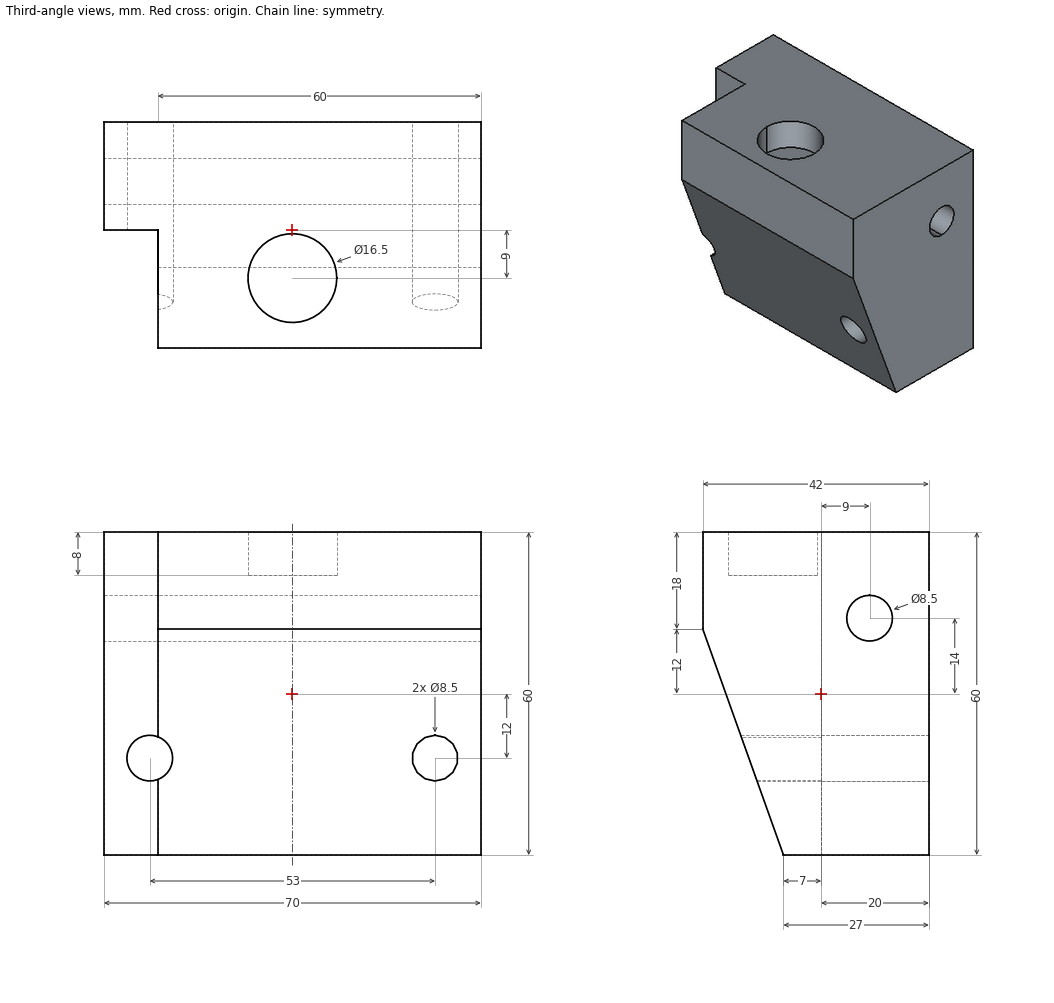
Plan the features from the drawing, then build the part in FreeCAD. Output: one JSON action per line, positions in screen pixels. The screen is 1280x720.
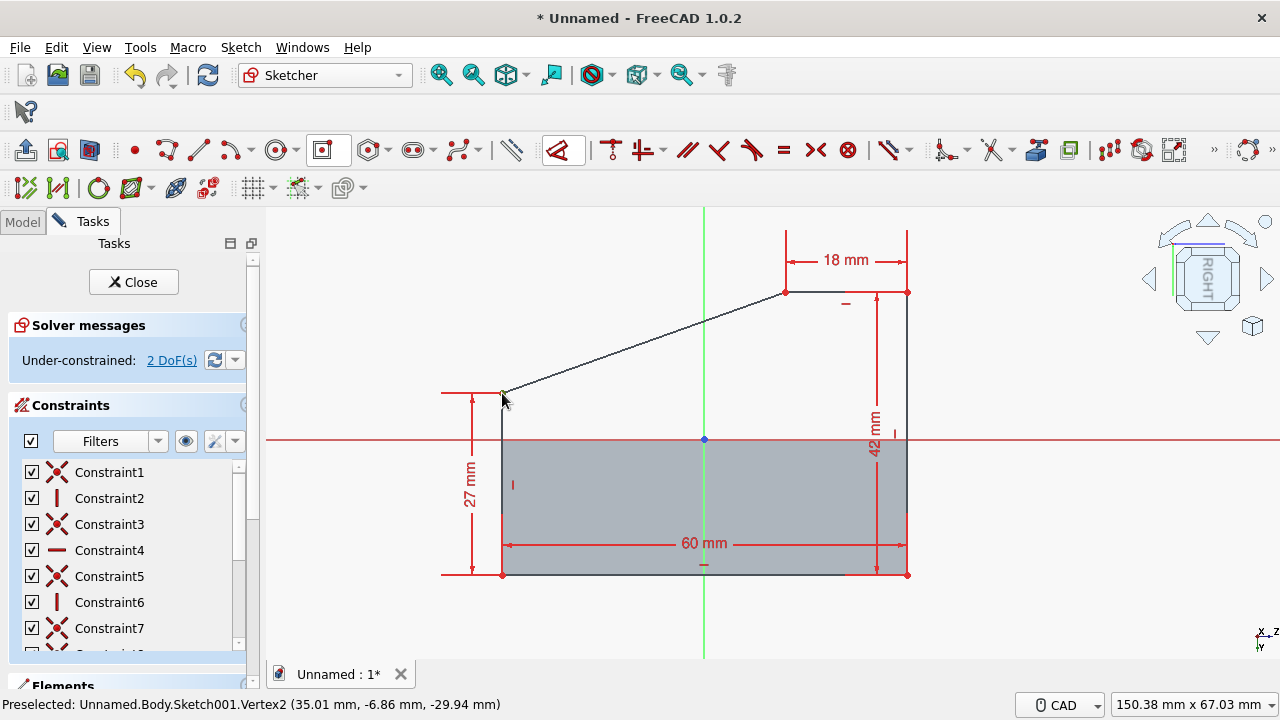
{"action": "key", "text": "i"}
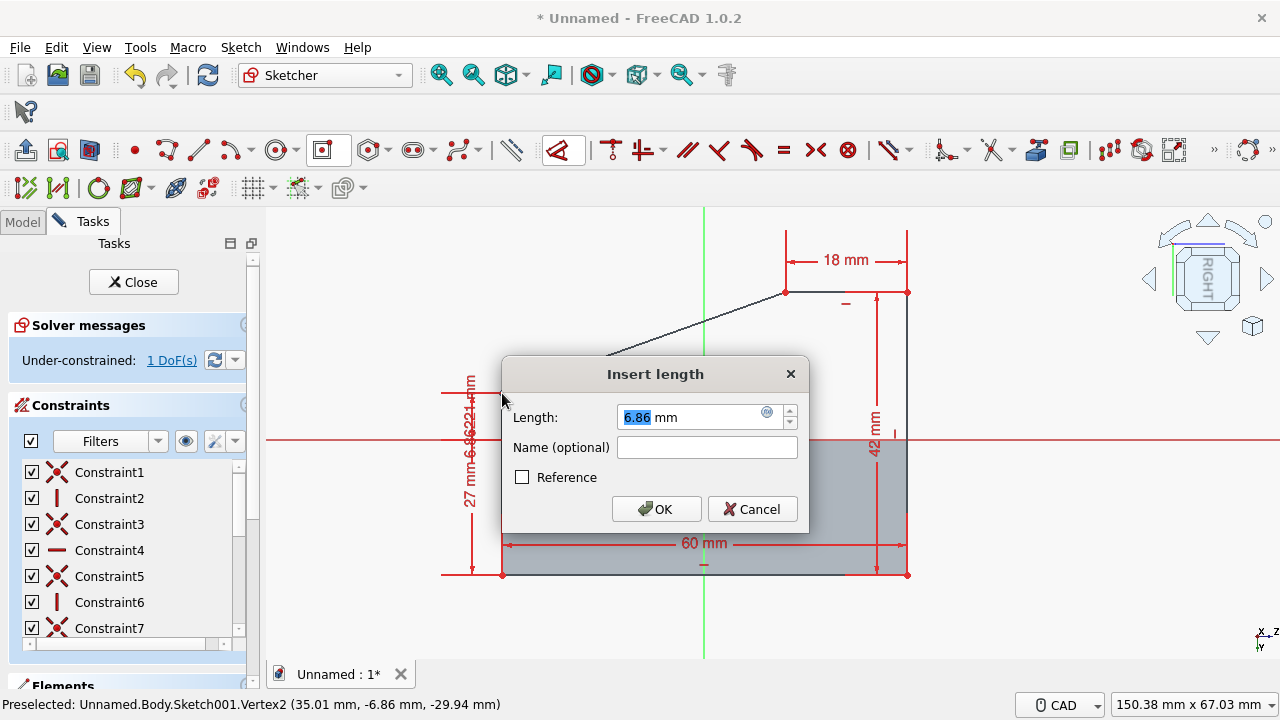
{"action": "type", "text": "7"}
{"action": "key", "text": "Return"}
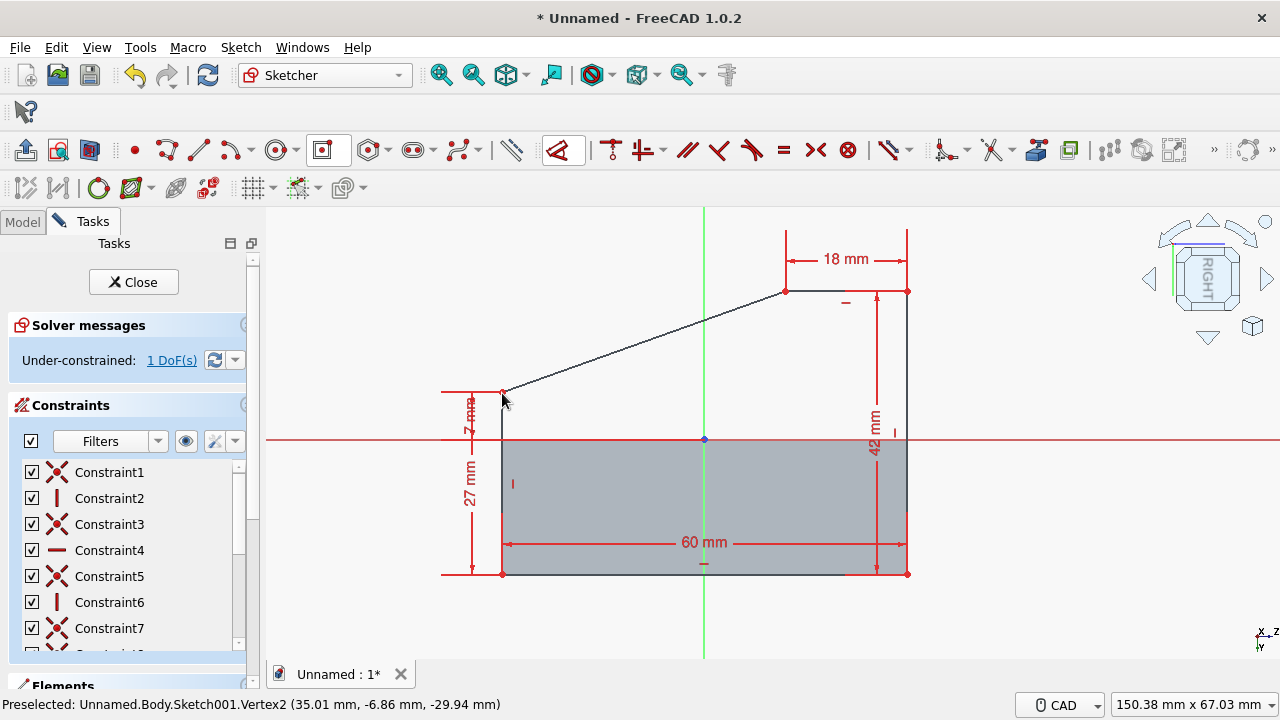
{"action": "left_click", "coordinate": [786, 291]}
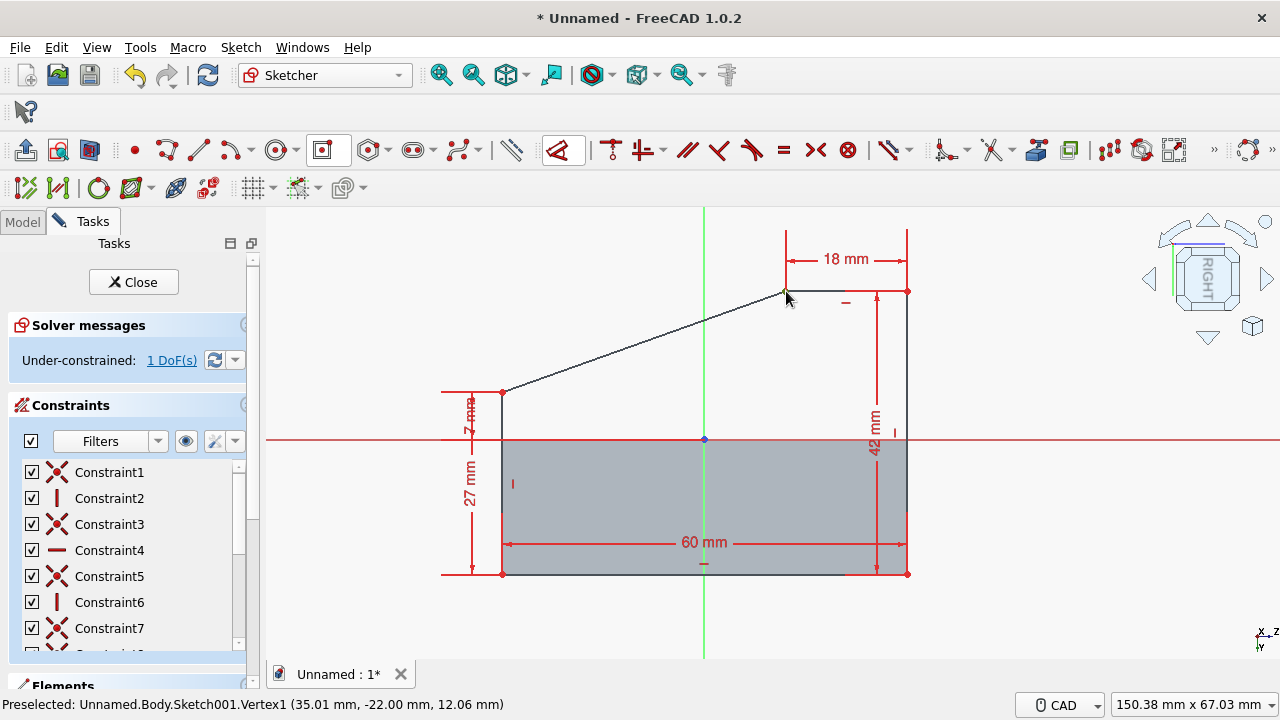
{"action": "left_click", "coordinate": [580, 150]}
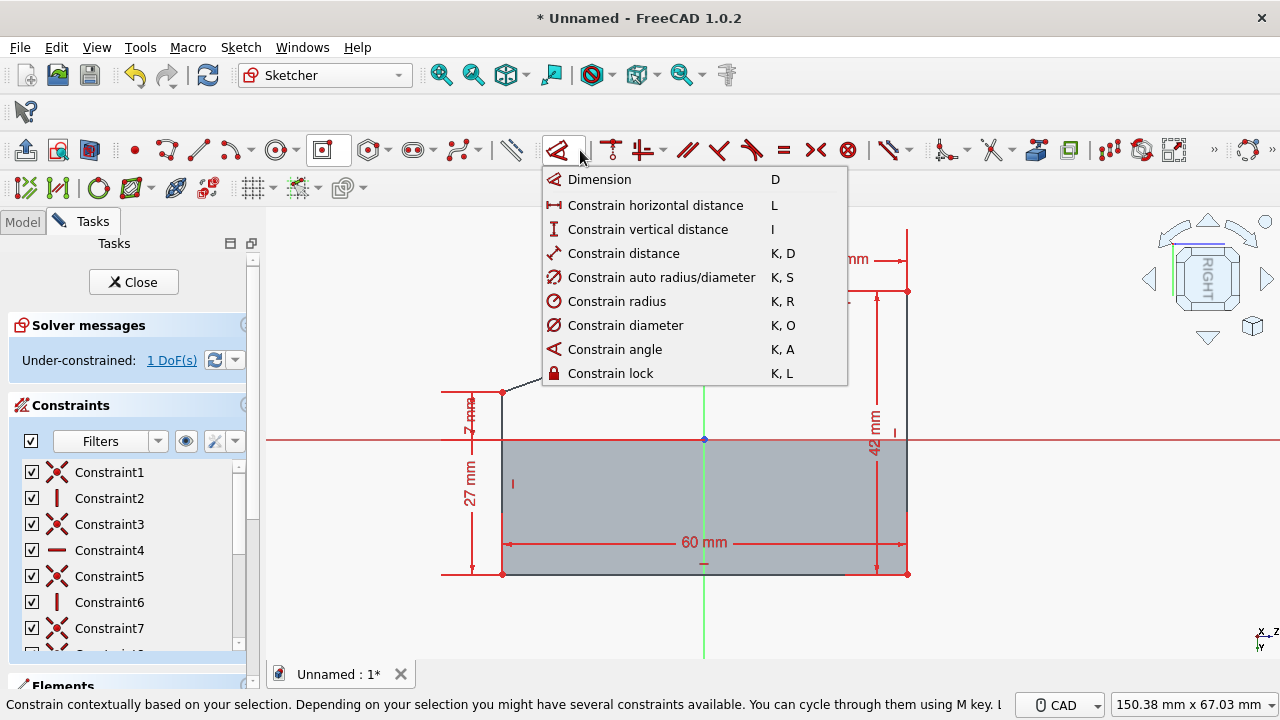
{"action": "left_click", "coordinate": [695, 205]}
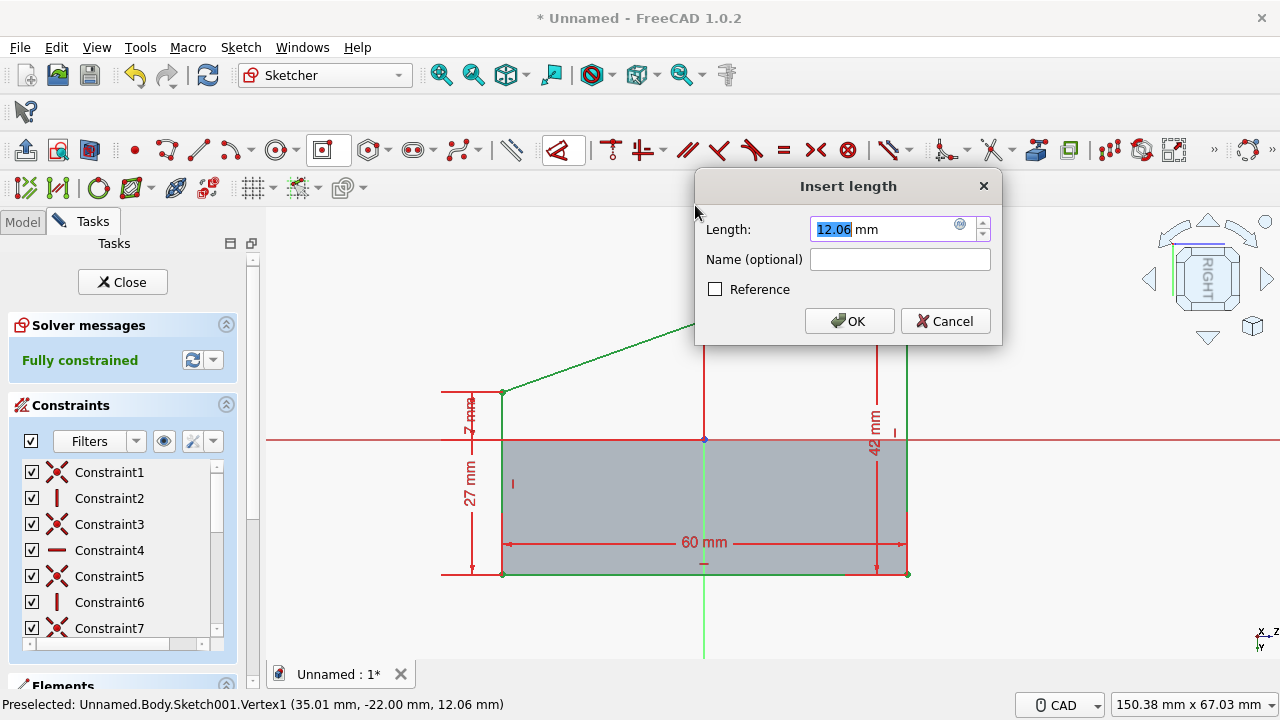
{"action": "type", "text": "12"}
{"action": "key", "text": "Return"}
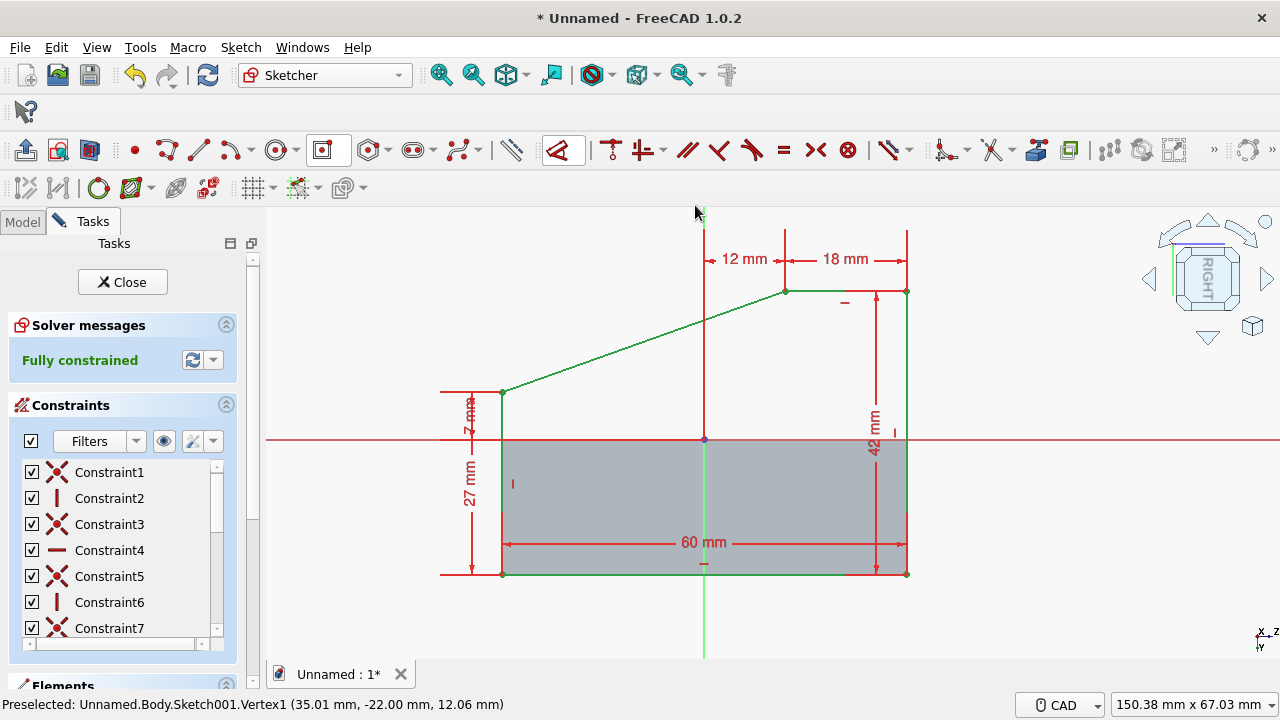
{"action": "left_click", "coordinate": [123, 282]}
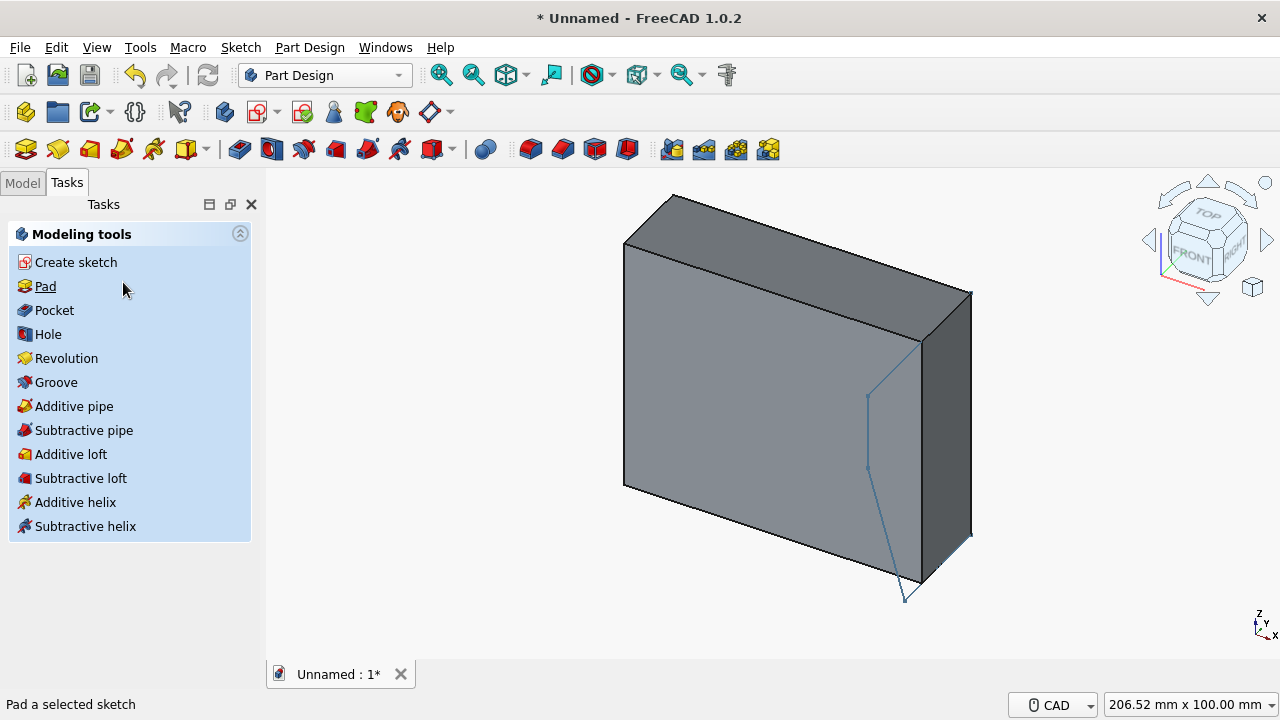
{"action": "left_click", "coordinate": [26, 150]}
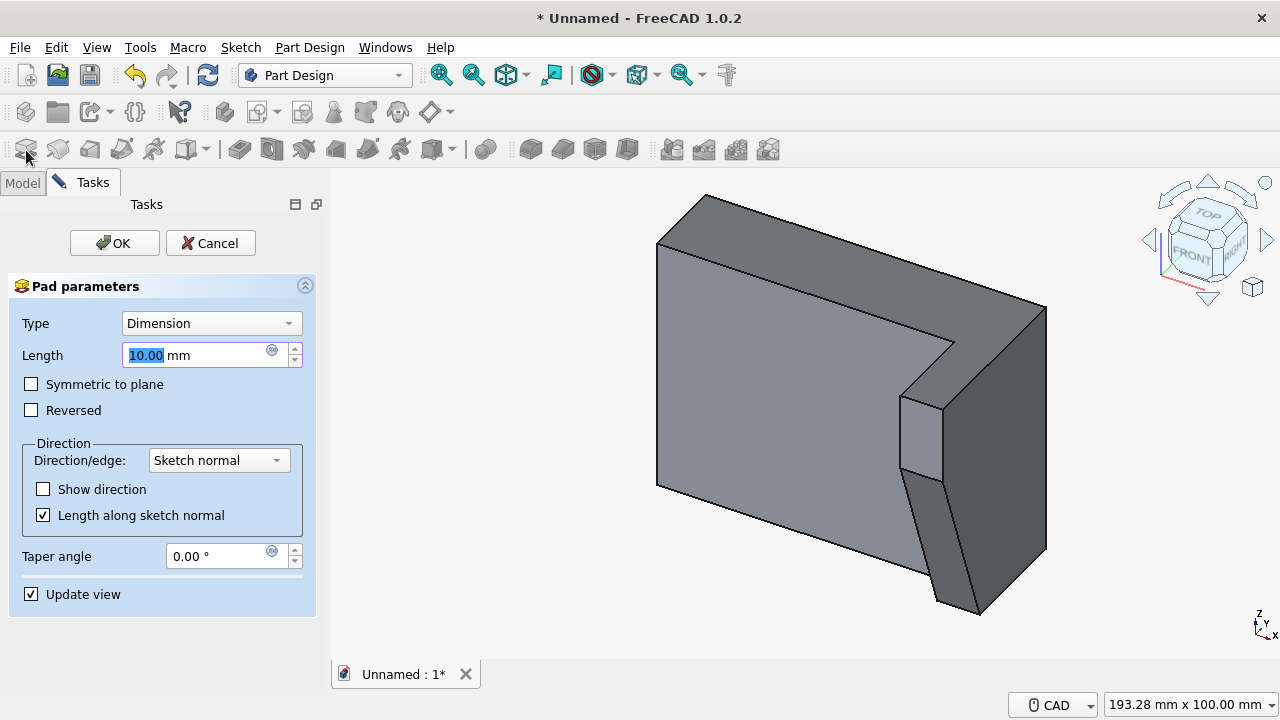
{"action": "type", "text": "60"}
{"action": "key", "text": "Tab"}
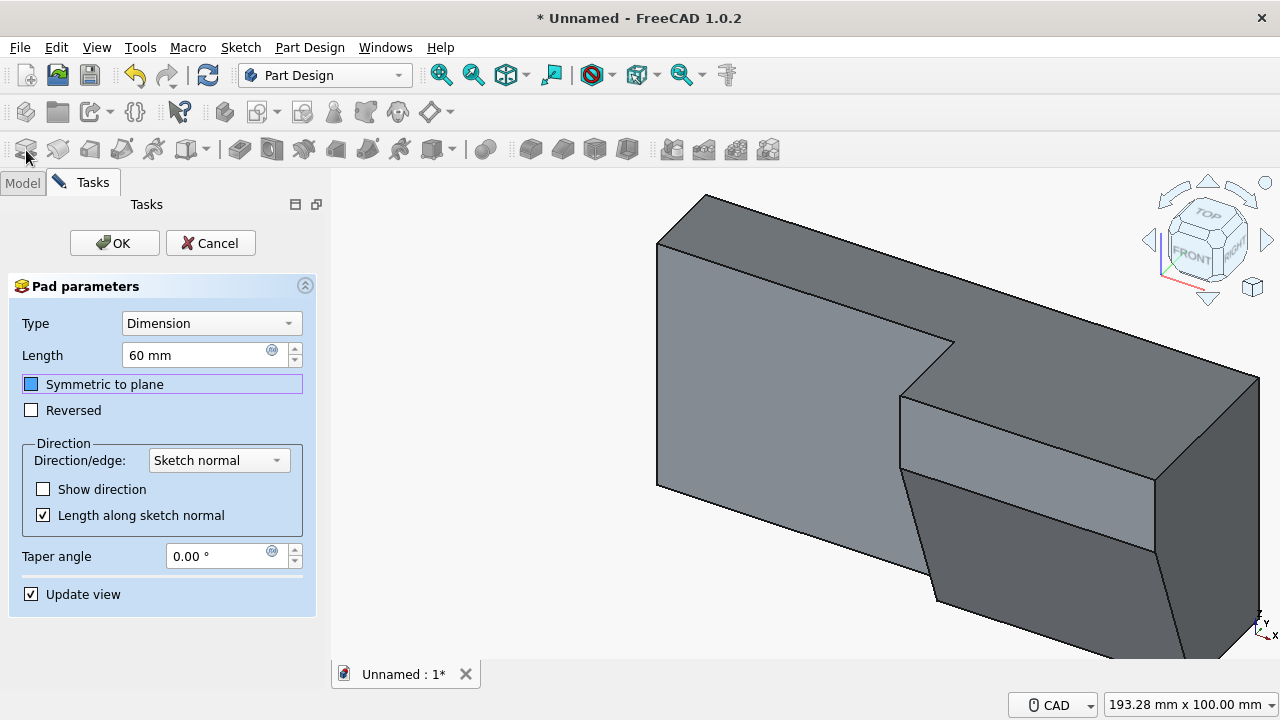
{"action": "left_click", "coordinate": [30, 410]}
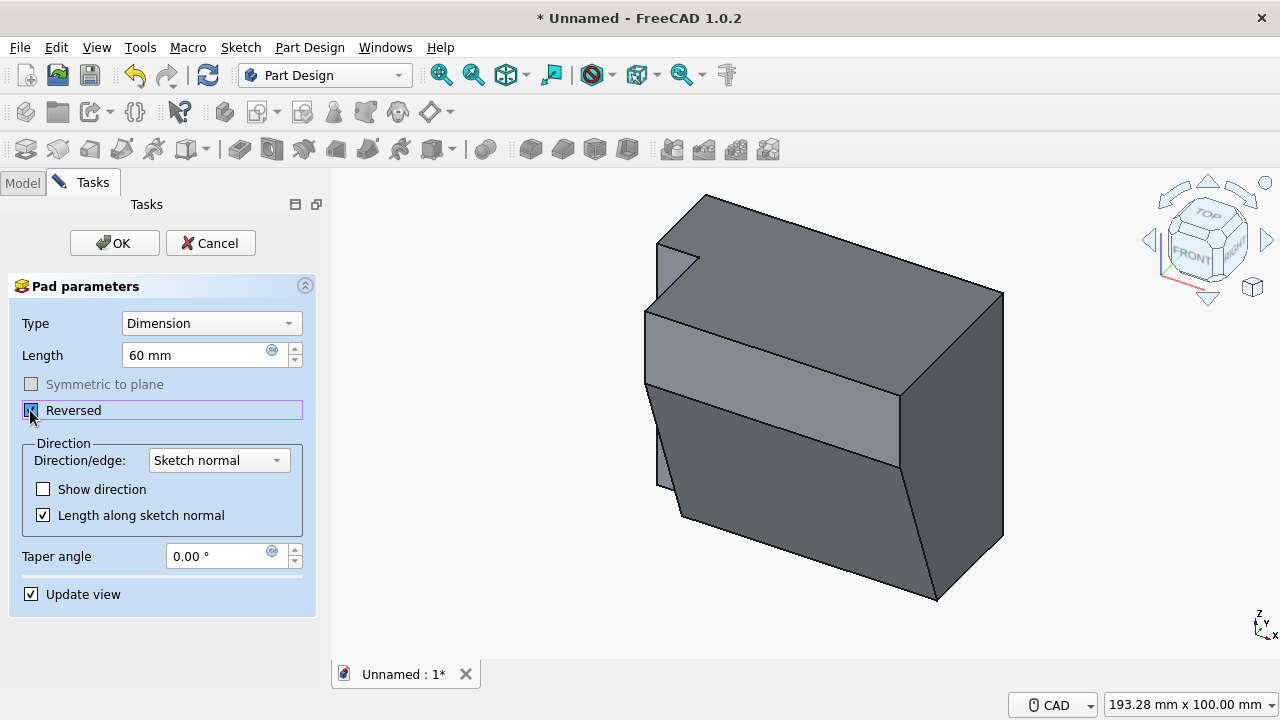
{"action": "left_click", "coordinate": [115, 243]}